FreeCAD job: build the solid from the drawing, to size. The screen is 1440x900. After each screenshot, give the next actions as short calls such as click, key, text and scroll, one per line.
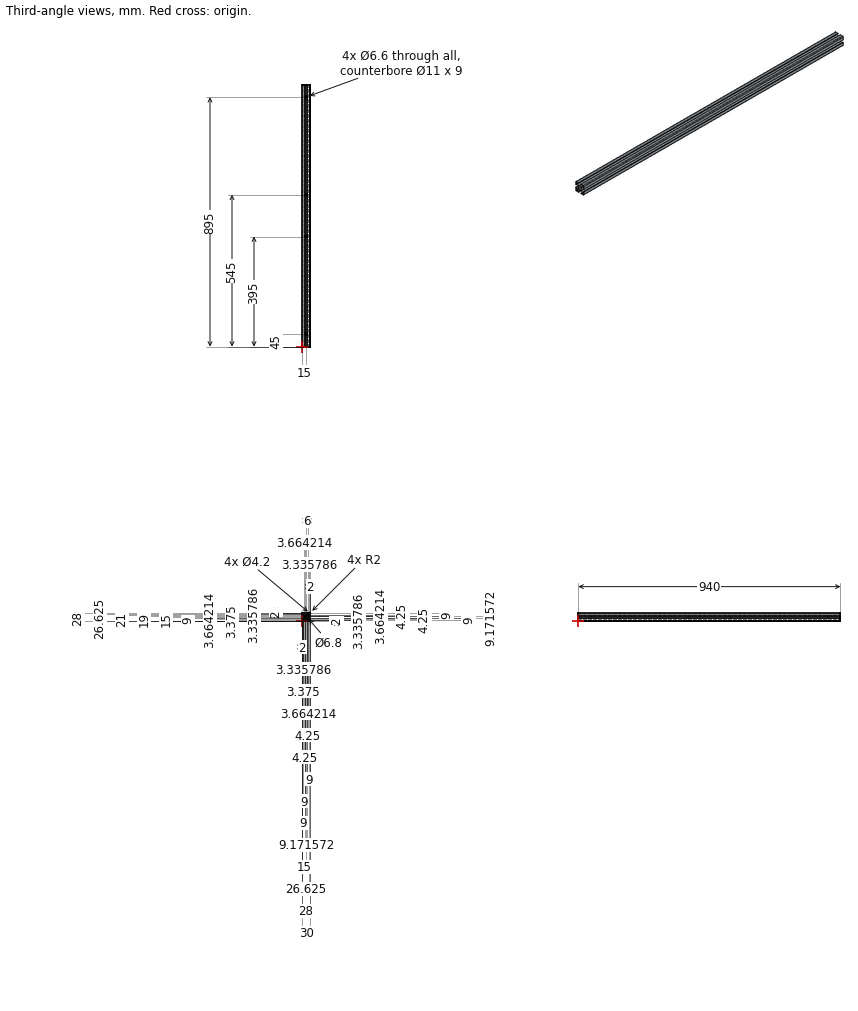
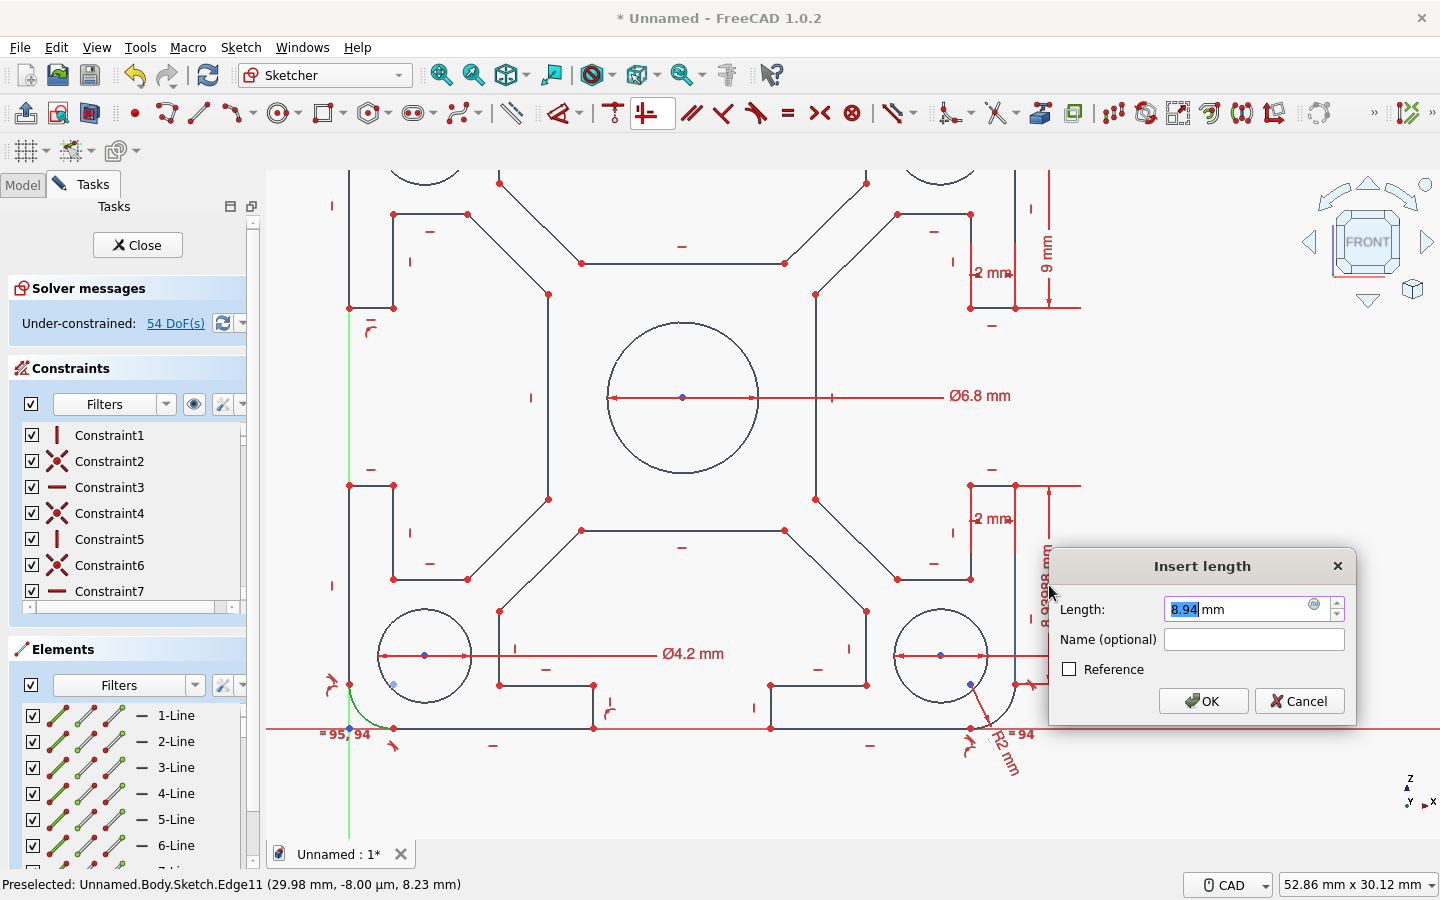
text(9)
key(Return)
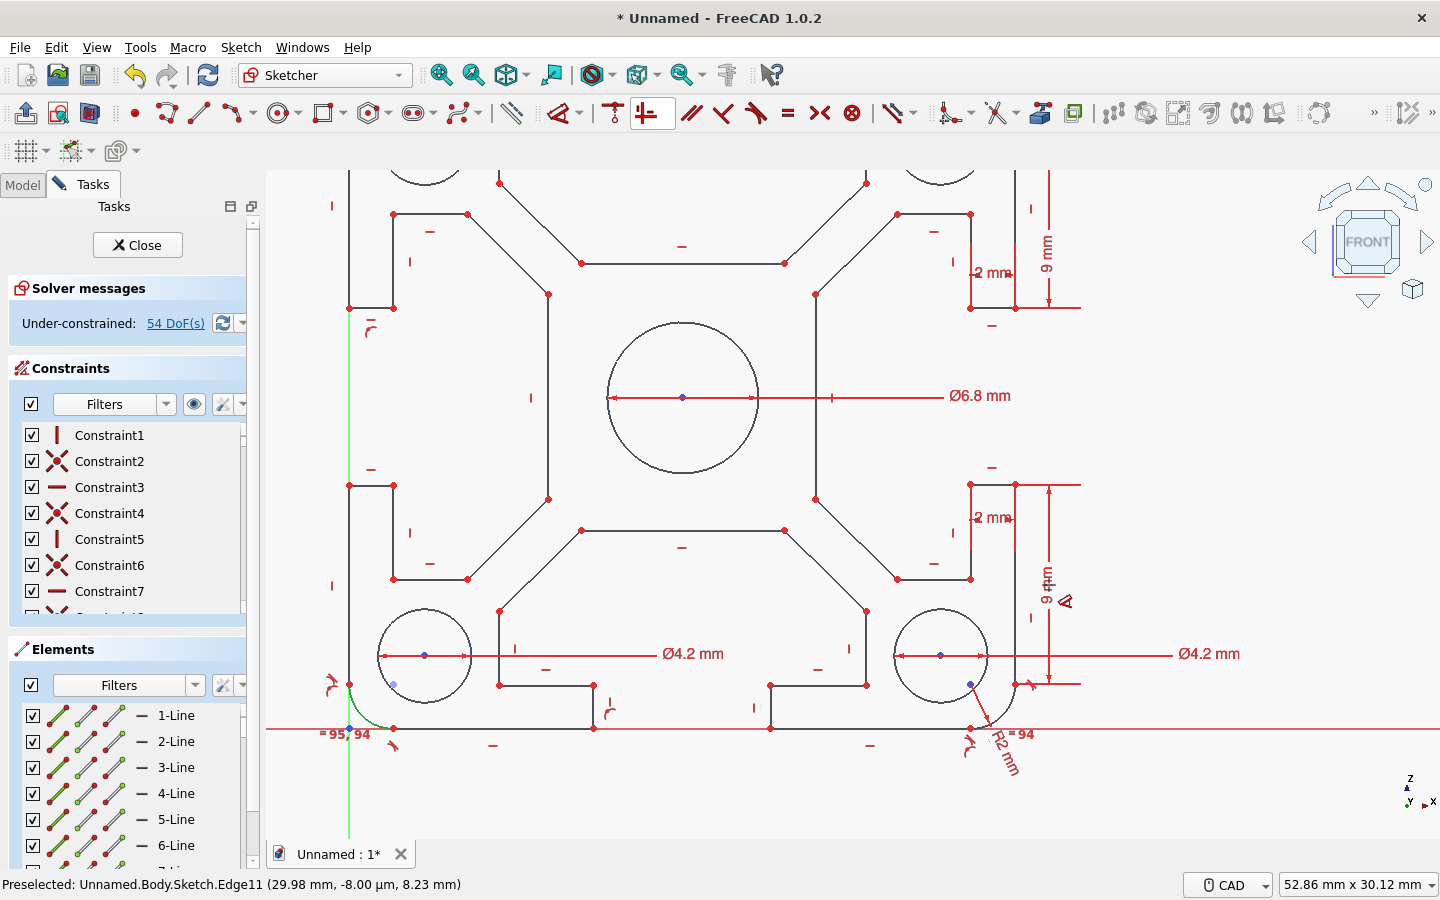
click(911, 729)
click(871, 763)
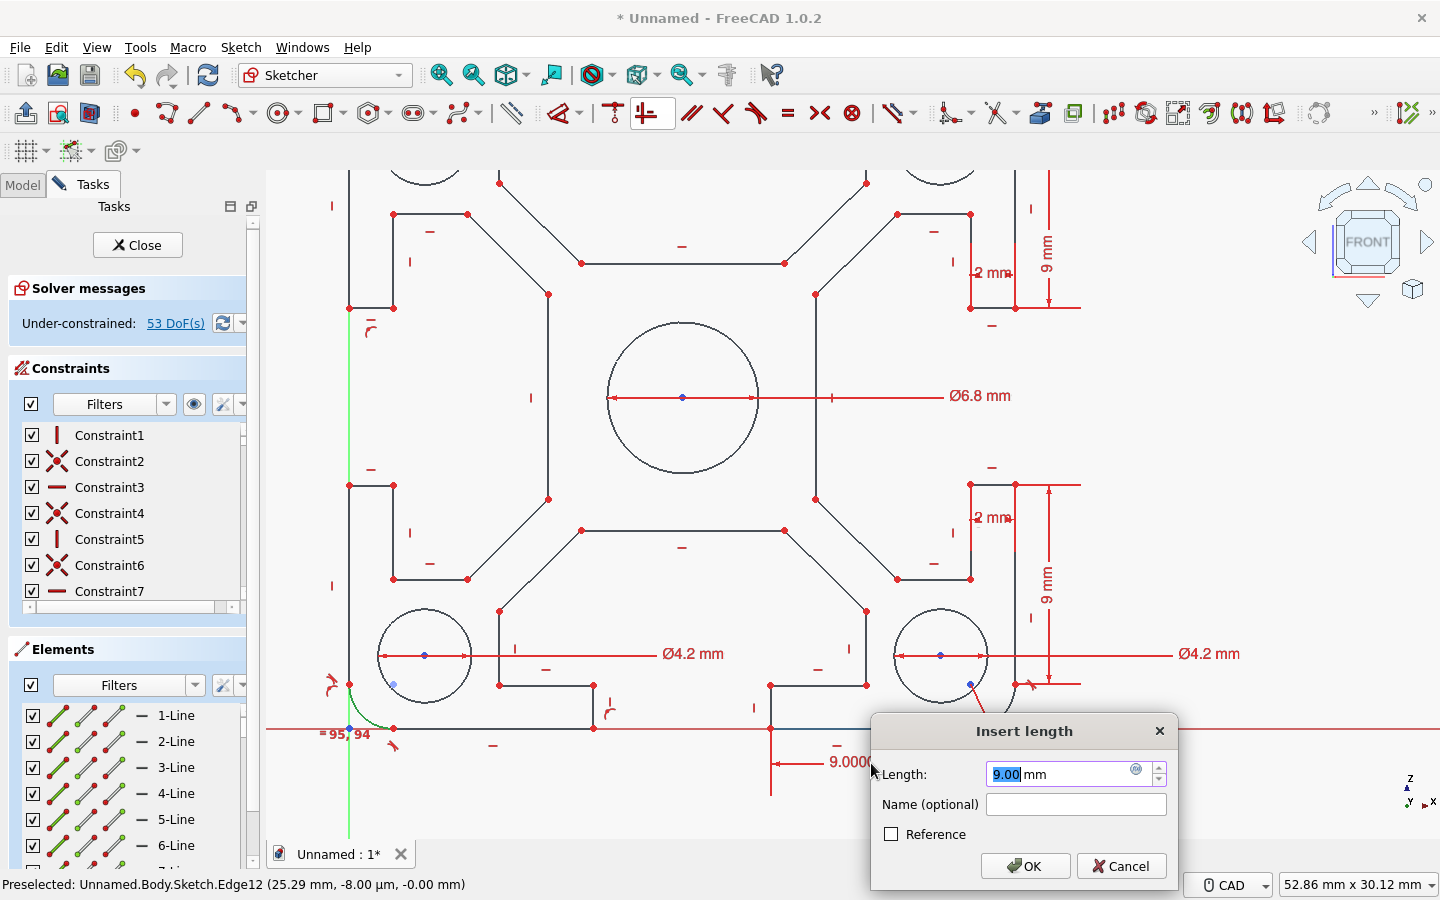
text(9)
key(Return)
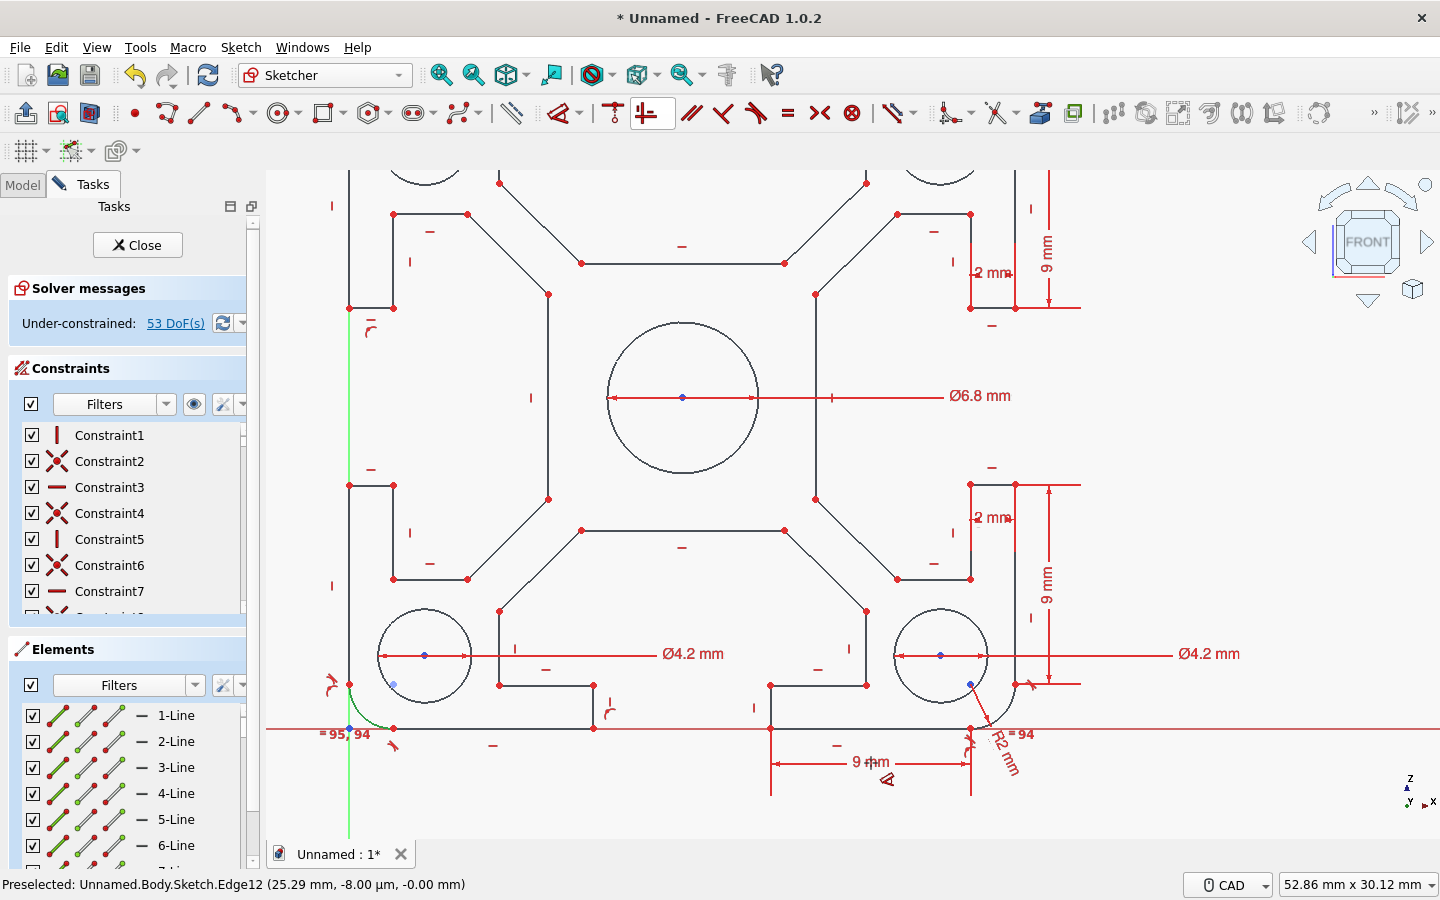
click(771, 716)
click(805, 707)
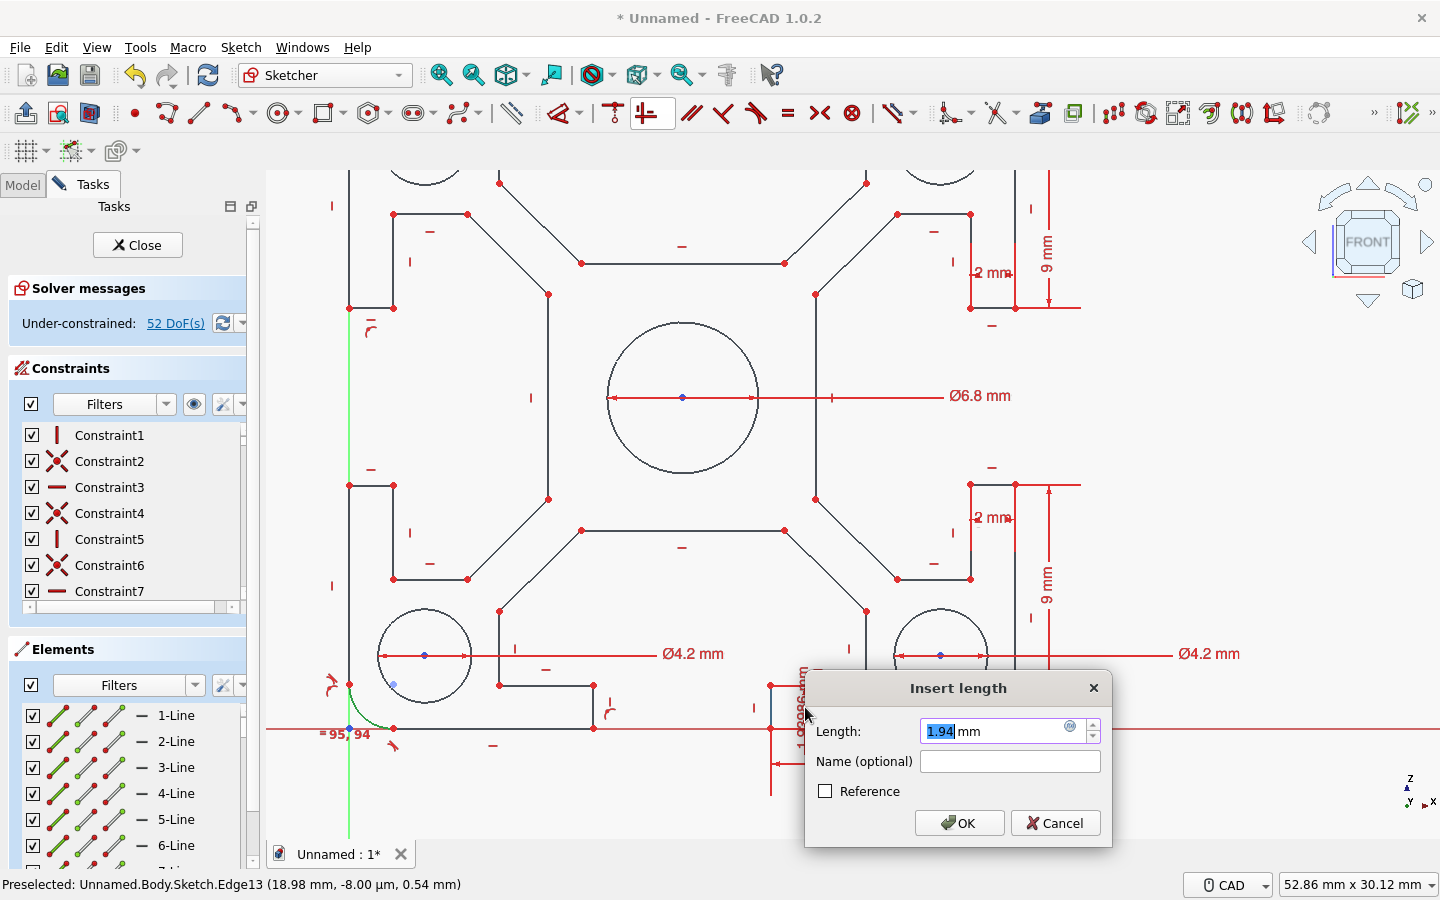
text(2)
key(Return)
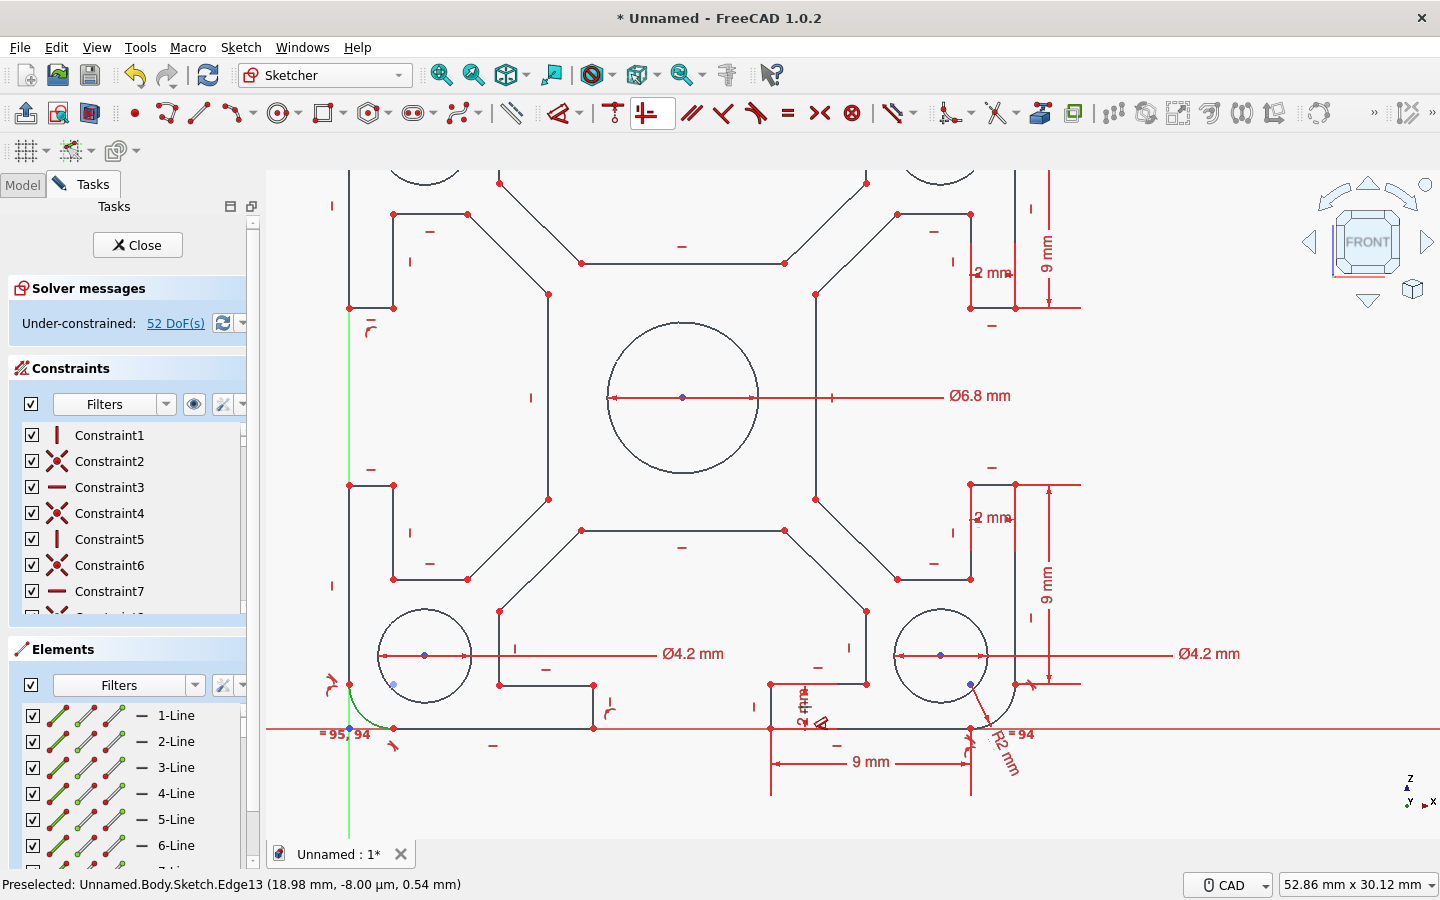
click(593, 699)
click(559, 707)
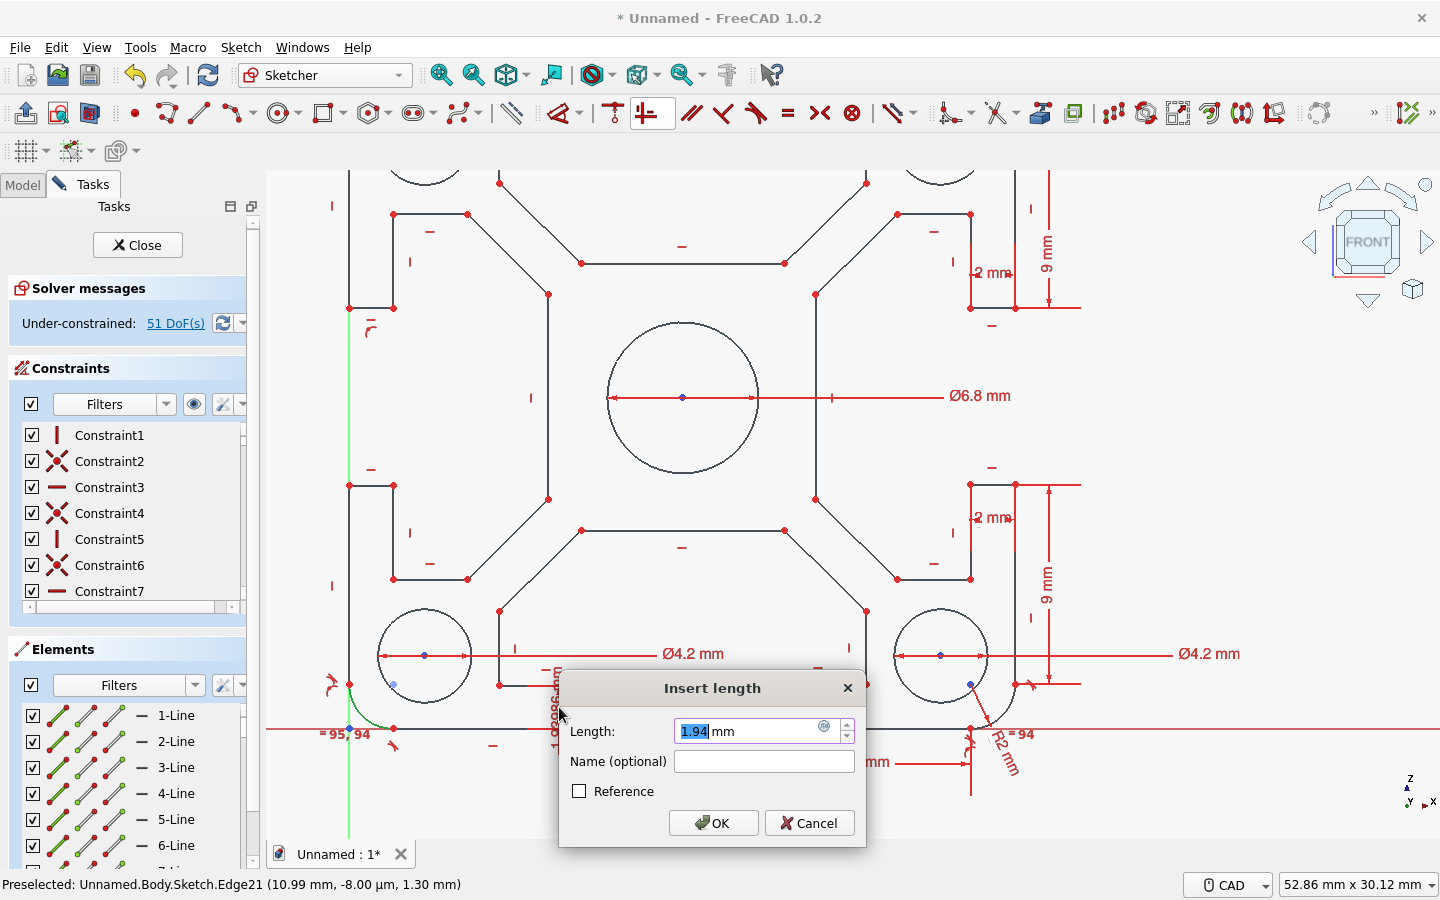
text(2)
key(Return)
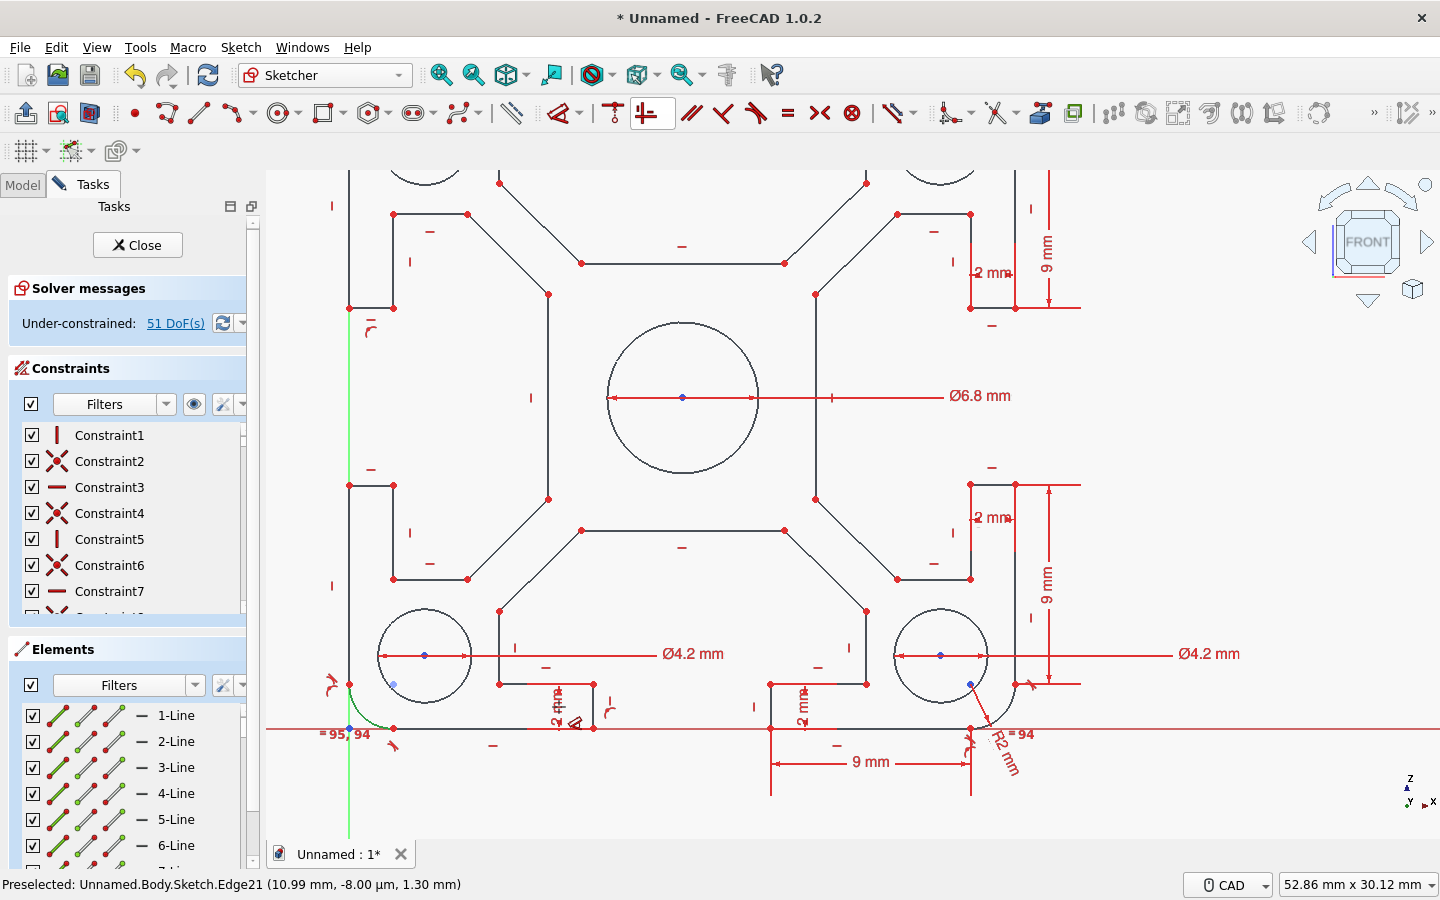
click(533, 729)
click(493, 763)